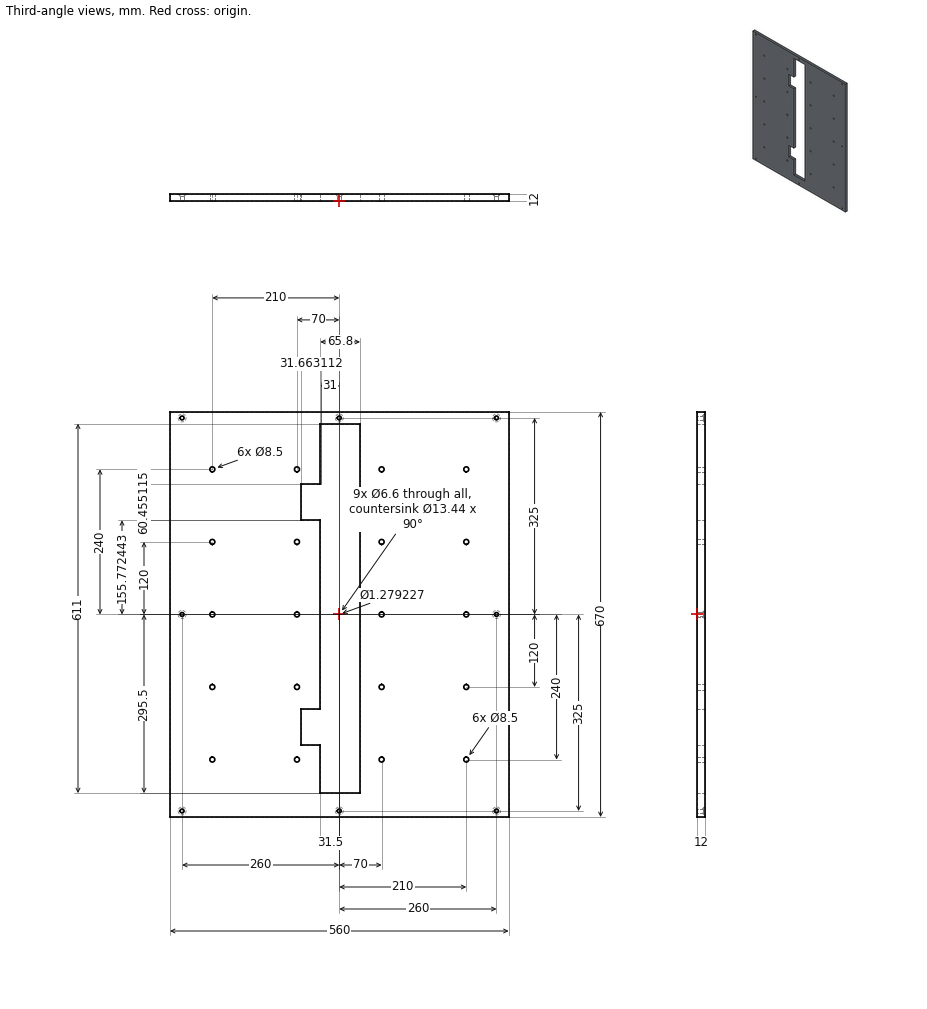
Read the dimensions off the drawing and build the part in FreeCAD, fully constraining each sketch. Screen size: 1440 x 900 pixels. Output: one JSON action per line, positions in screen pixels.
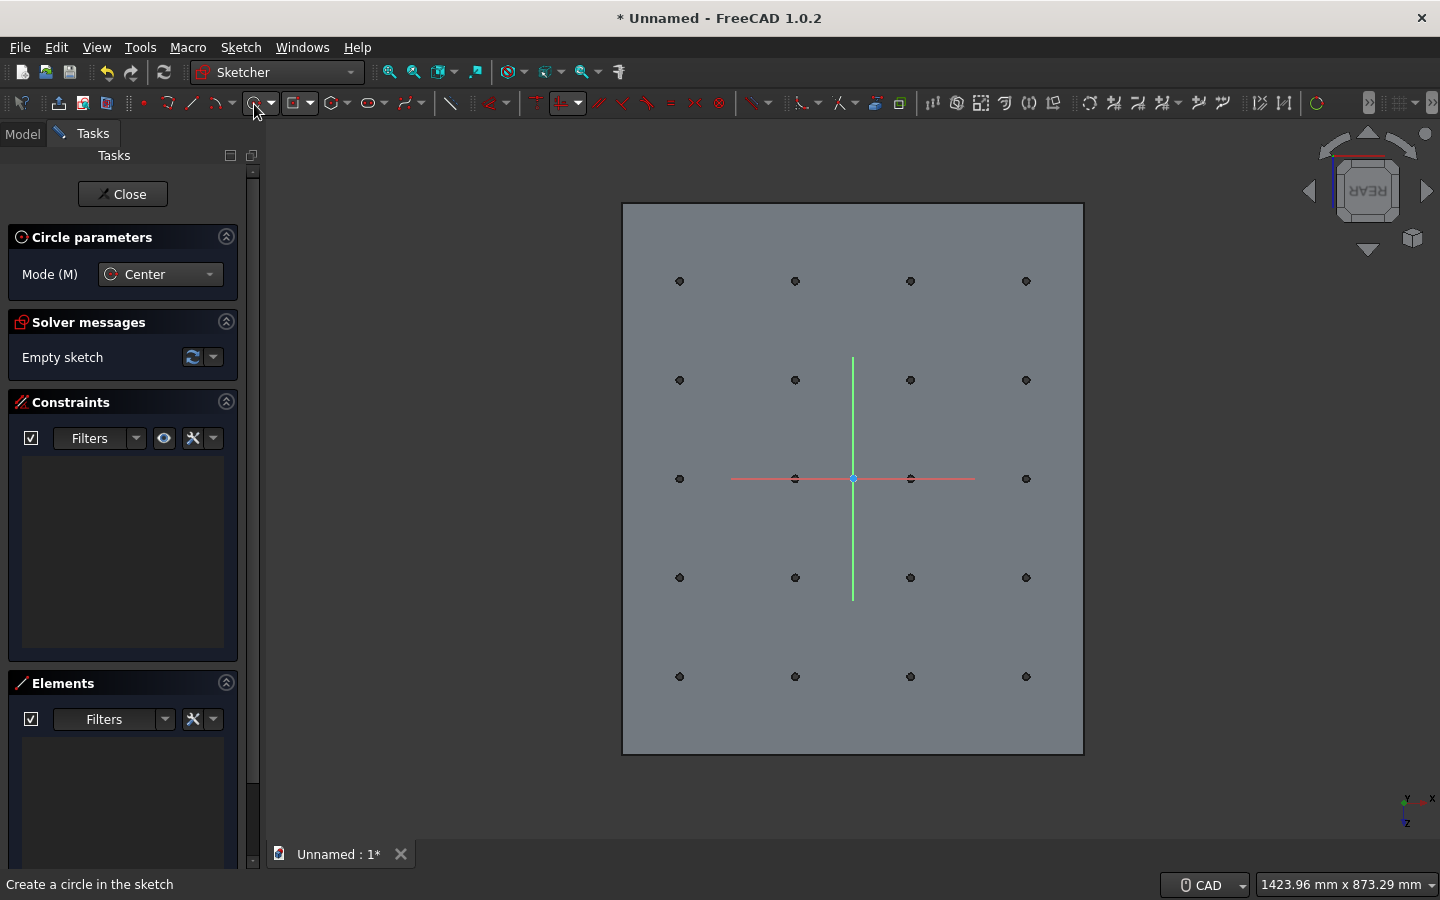
{"action": "scroll", "coordinate": [853, 479], "scroll_direction": "up", "scroll_amount": 11}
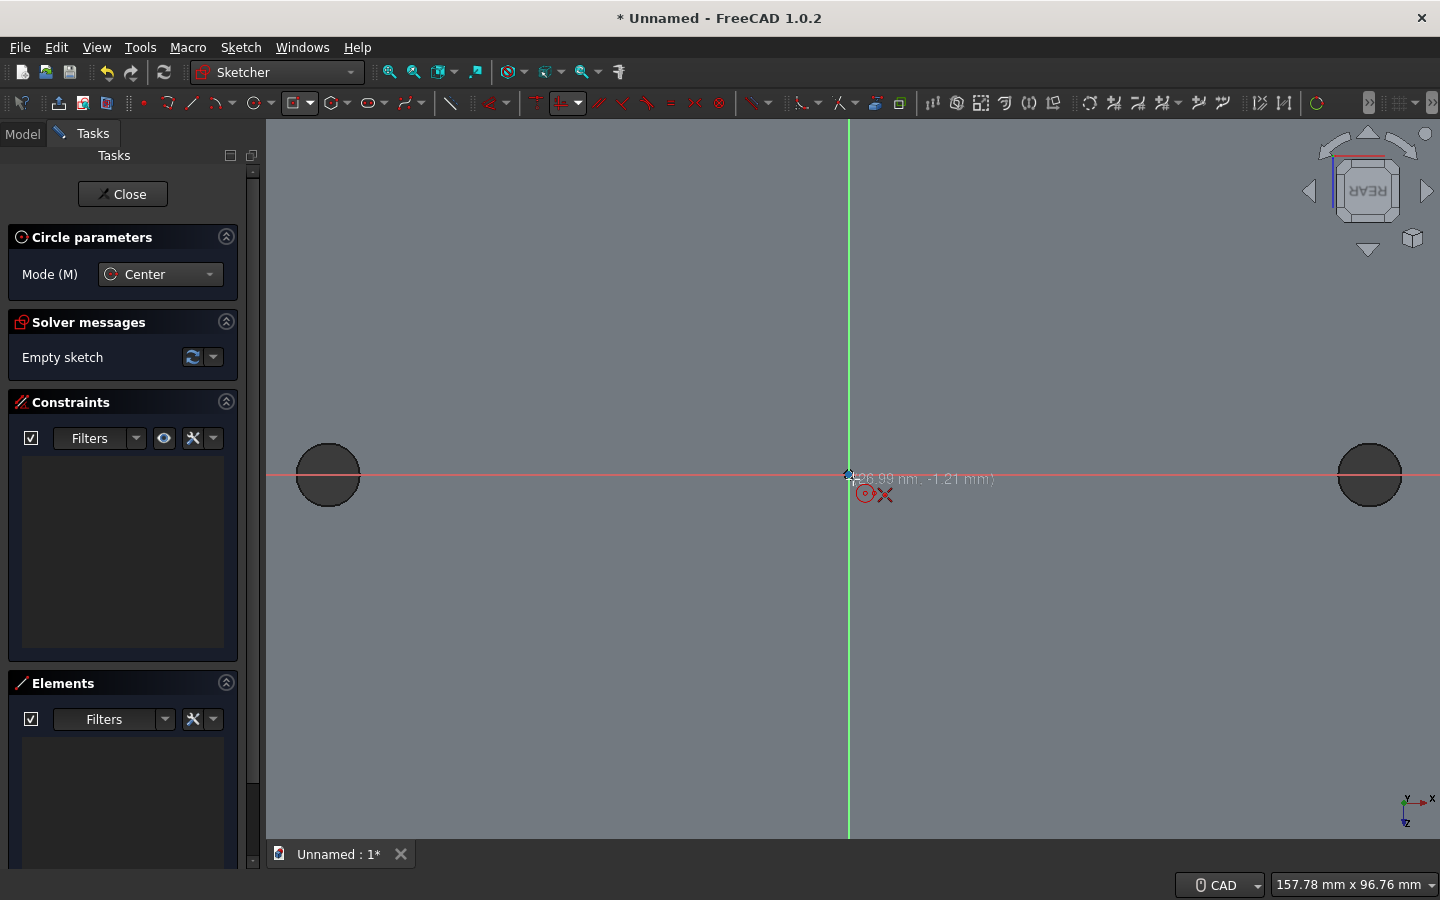
{"action": "scroll", "coordinate": [778, 479], "scroll_direction": "down", "scroll_amount": 12}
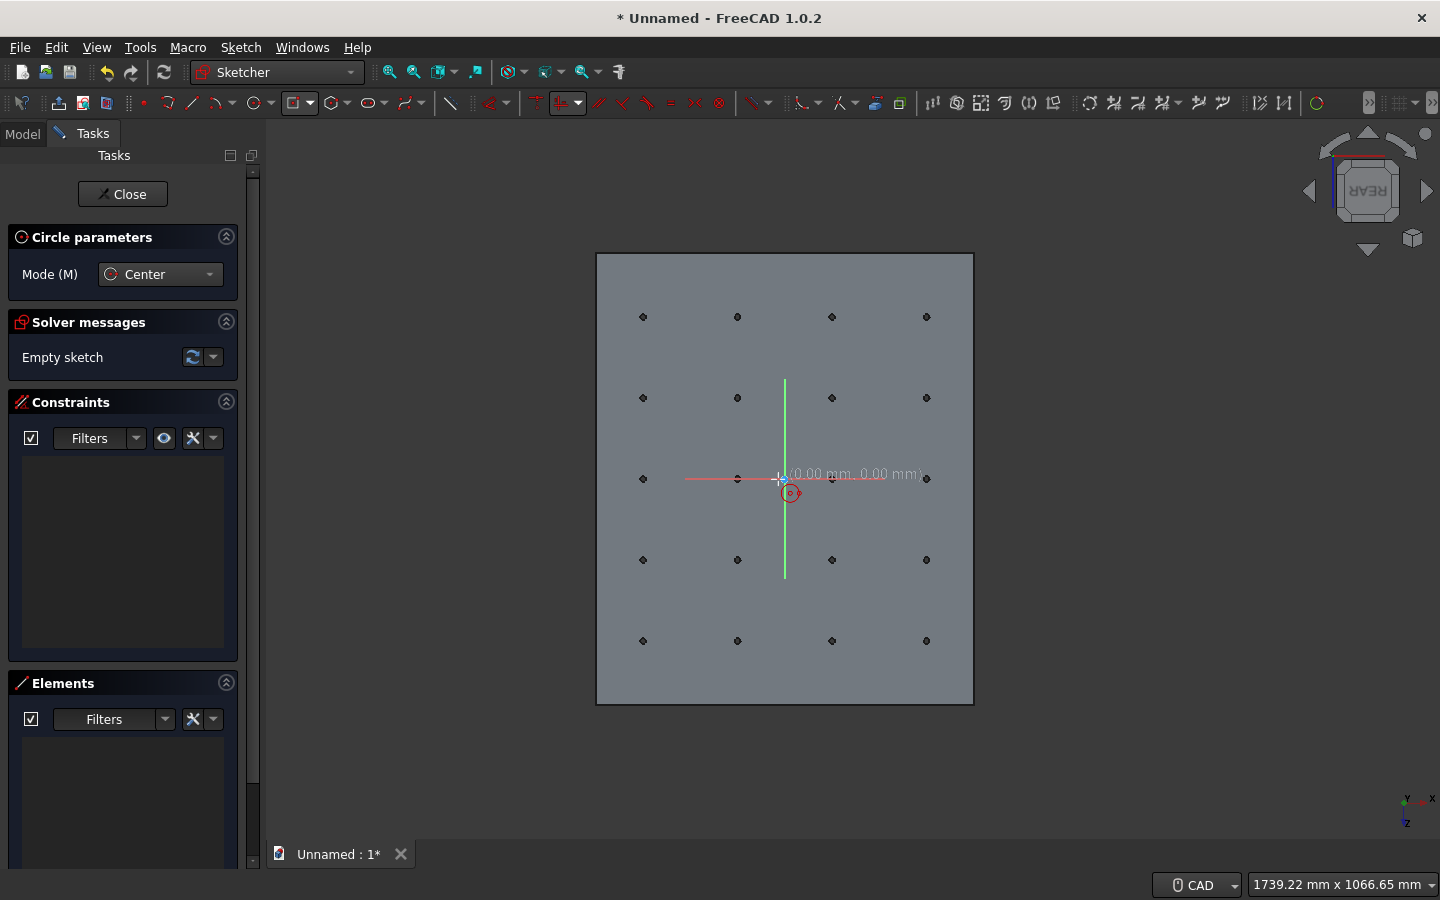
{"action": "left_click", "coordinate": [785, 479]}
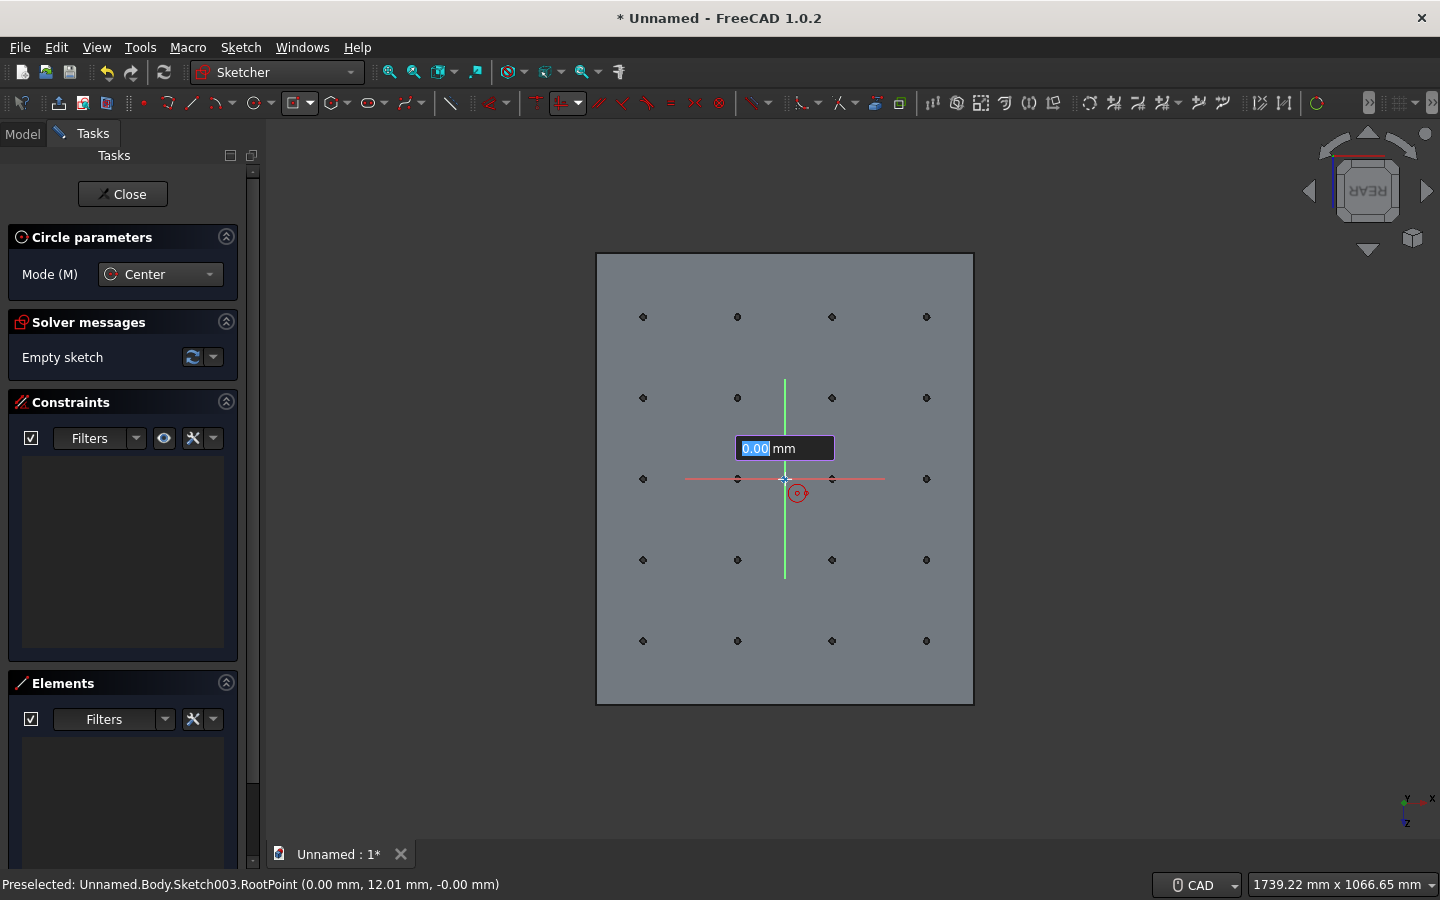
{"action": "scroll", "coordinate": [786, 478], "scroll_direction": "up", "scroll_amount": 12}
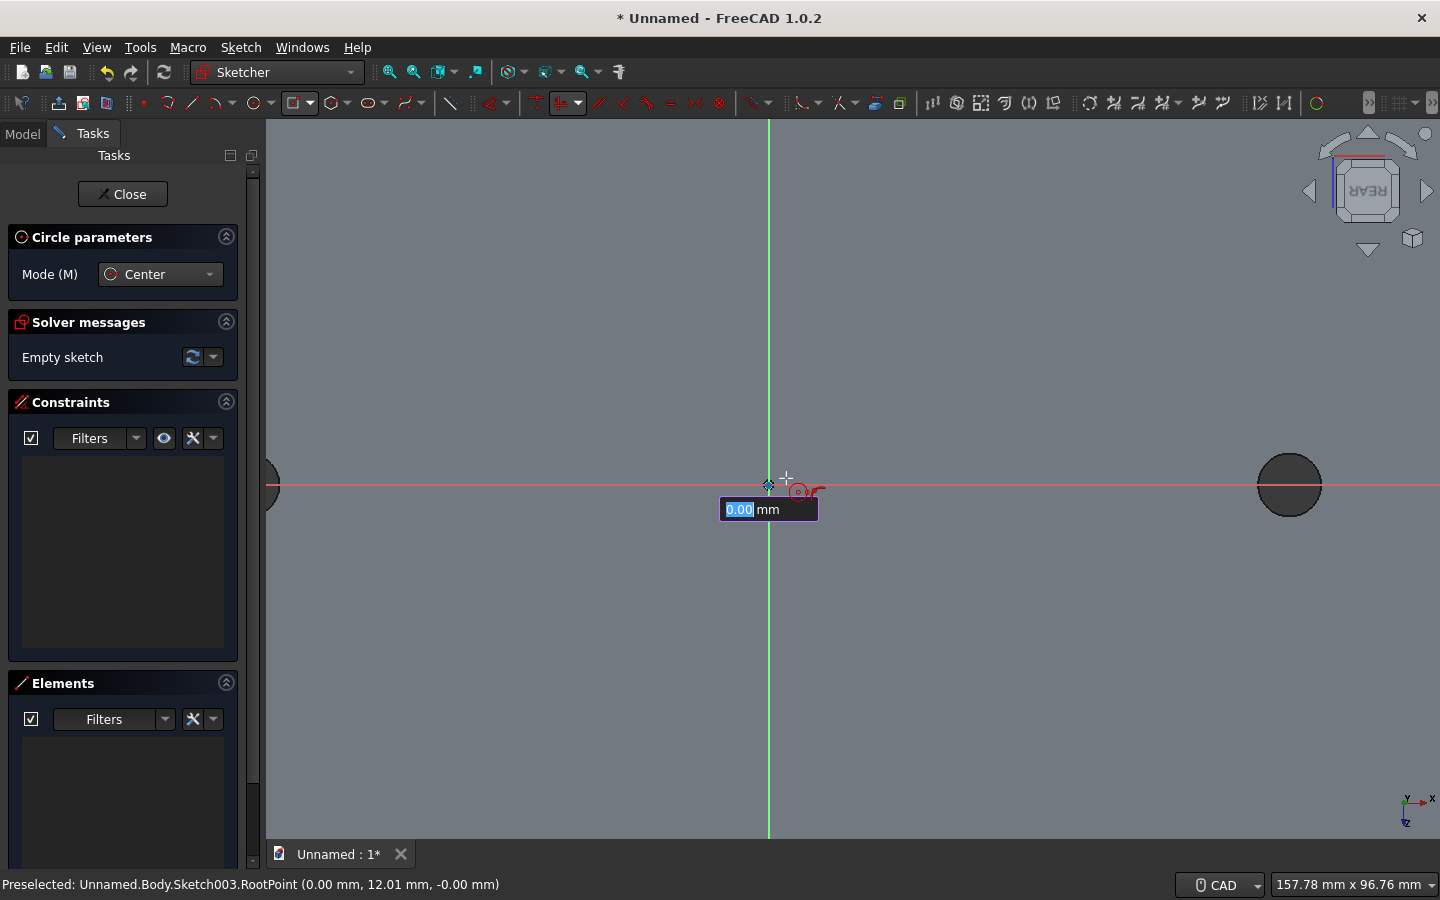
{"action": "left_click", "coordinate": [786, 468]}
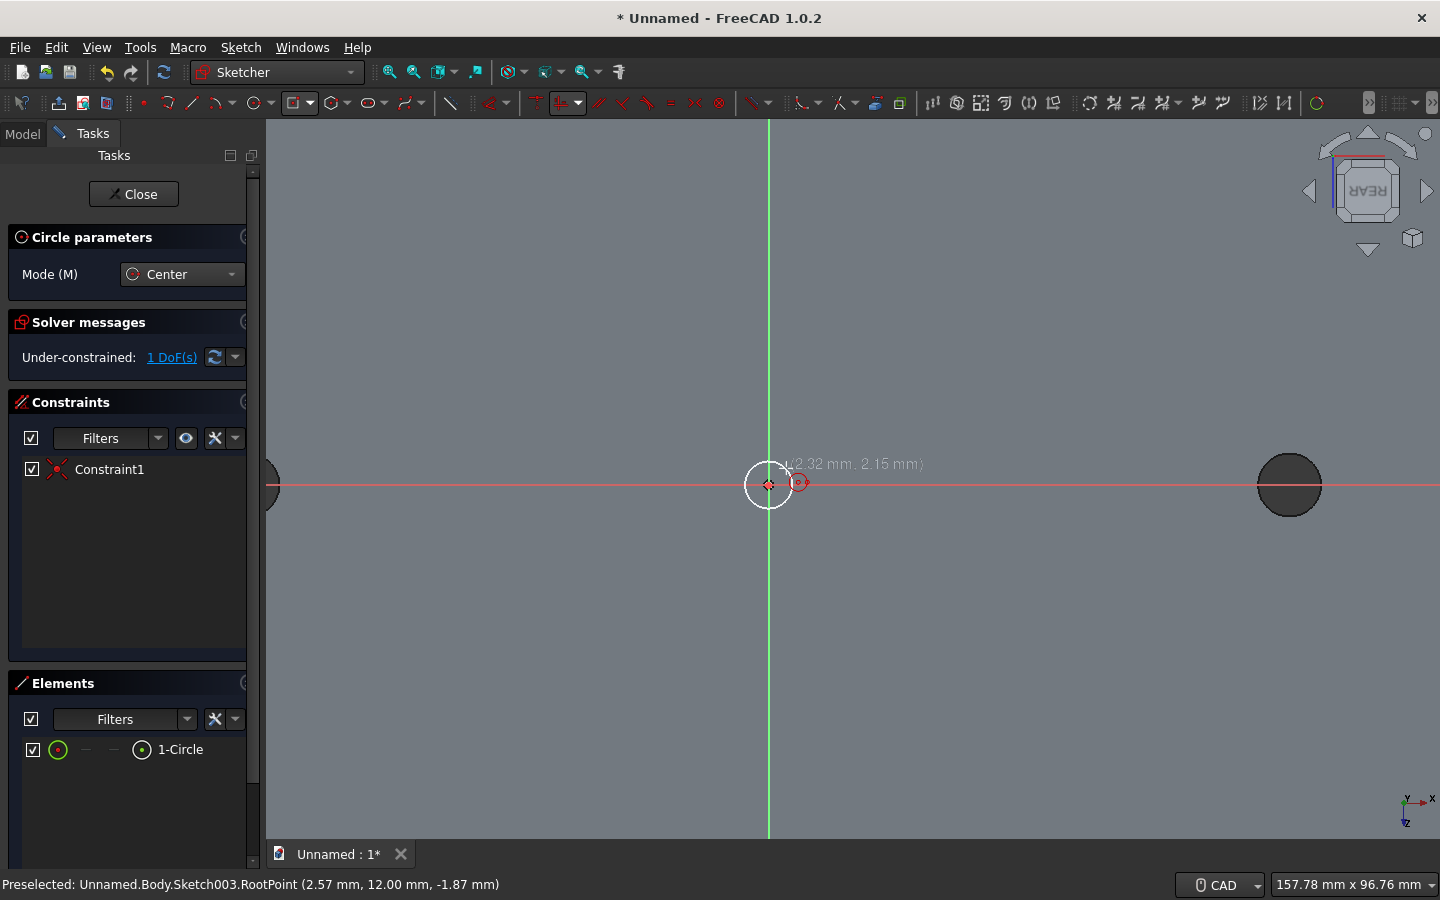
{"action": "scroll", "coordinate": [786, 478], "scroll_direction": "down", "scroll_amount": 12}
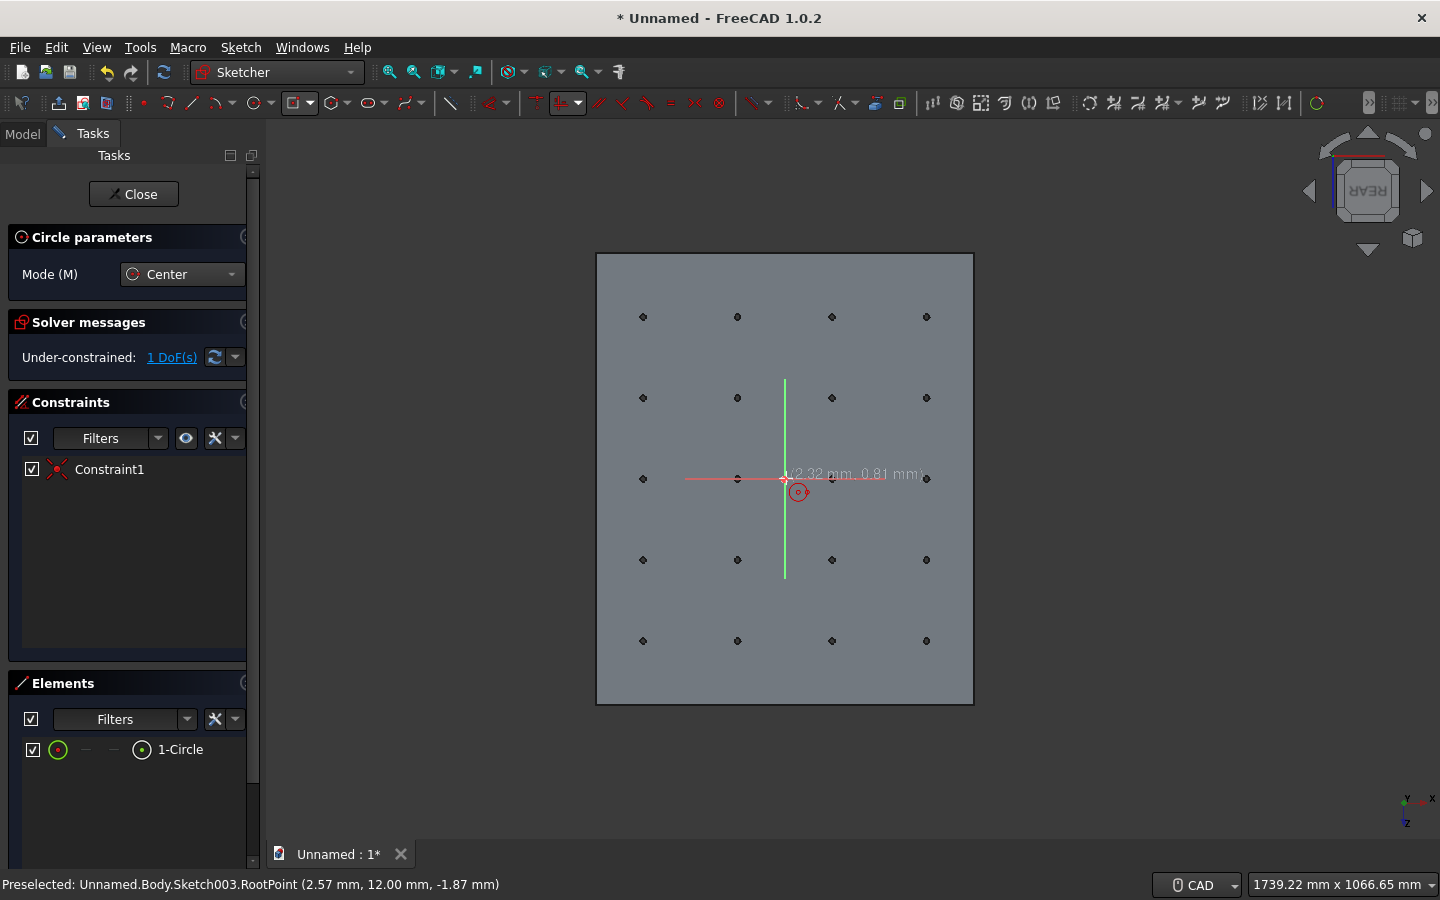
{"action": "scroll", "coordinate": [960, 479], "scroll_direction": "up", "scroll_amount": 12}